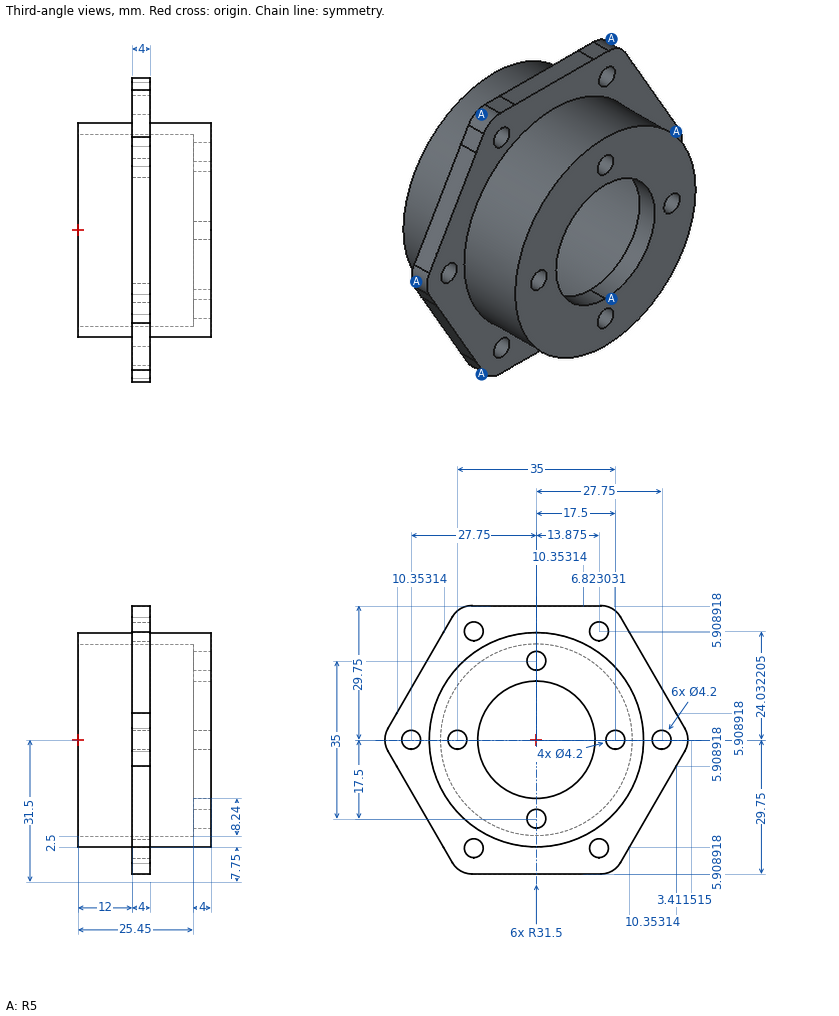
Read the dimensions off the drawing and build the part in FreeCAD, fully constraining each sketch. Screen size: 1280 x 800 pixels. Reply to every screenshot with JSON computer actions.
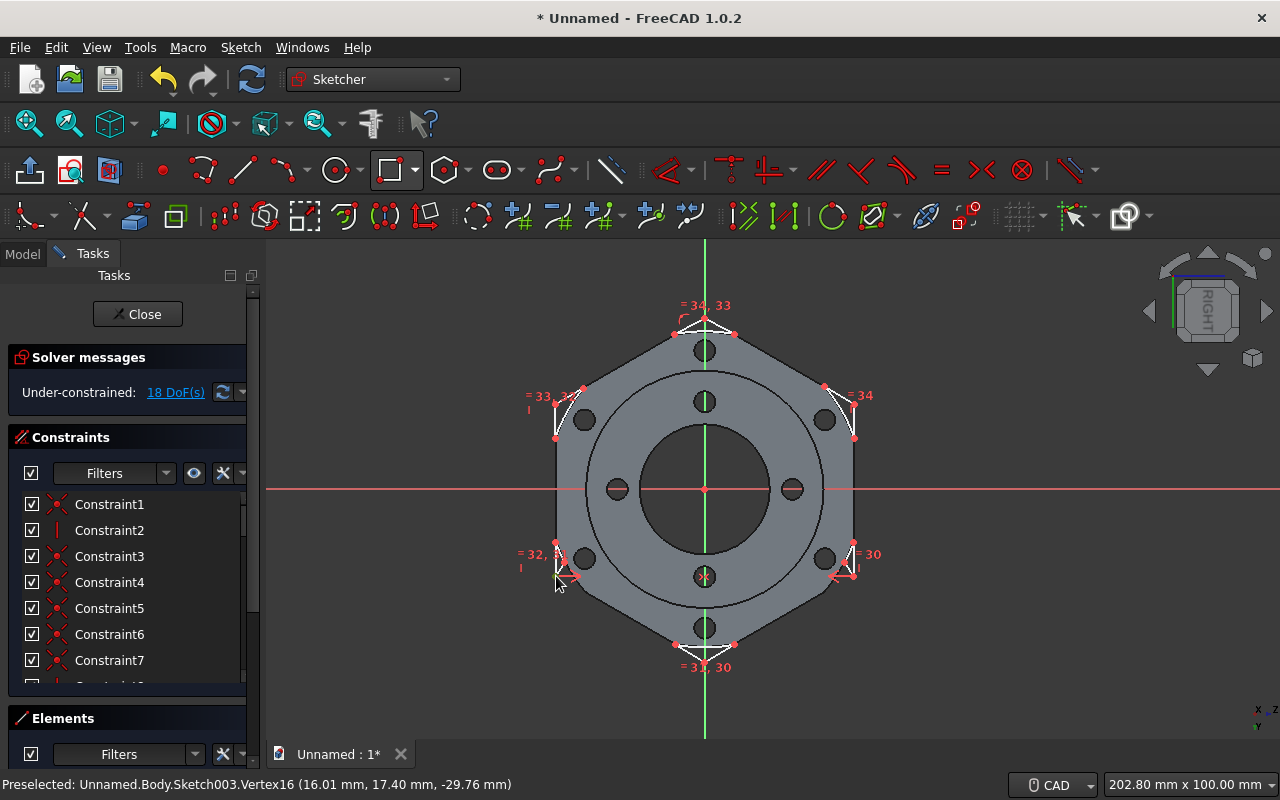
{"action": "left_click", "coordinate": [555, 405]}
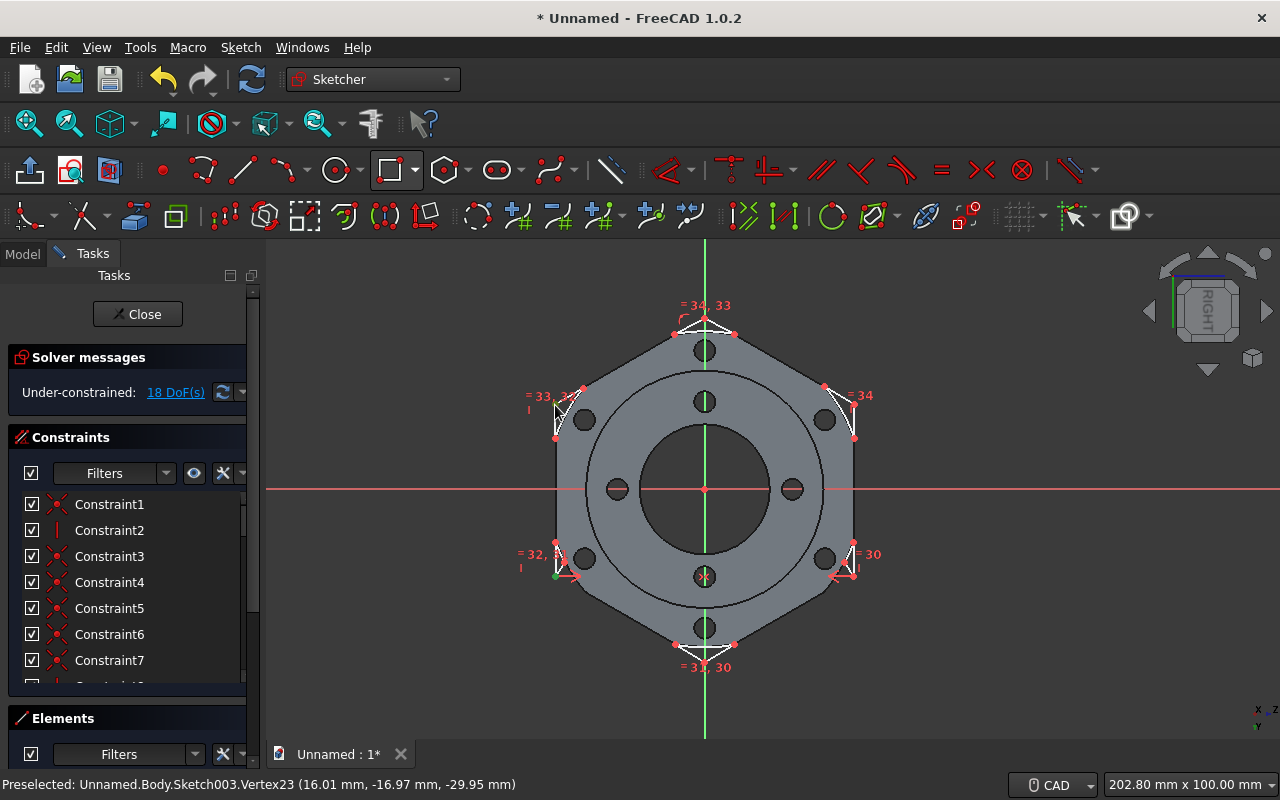
{"action": "left_click", "coordinate": [353, 489]}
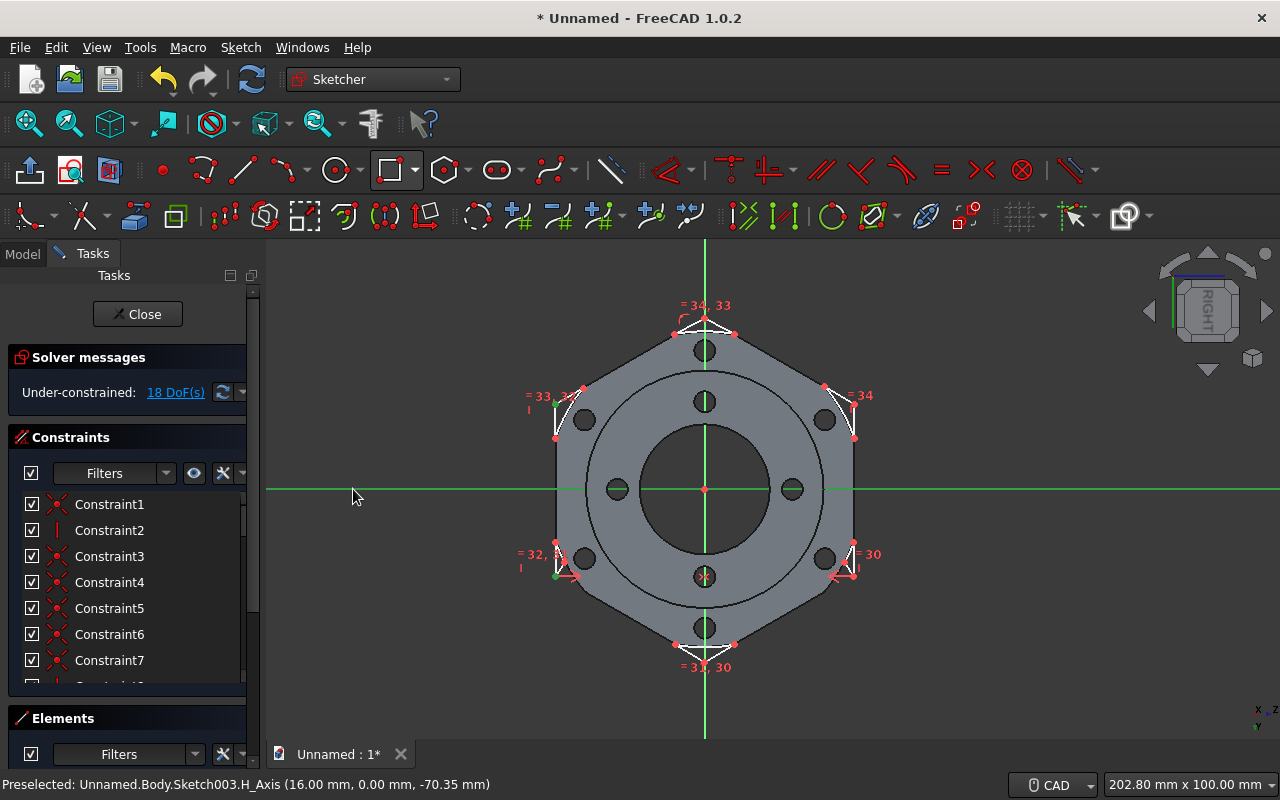
{"action": "left_click", "coordinate": [982, 170]}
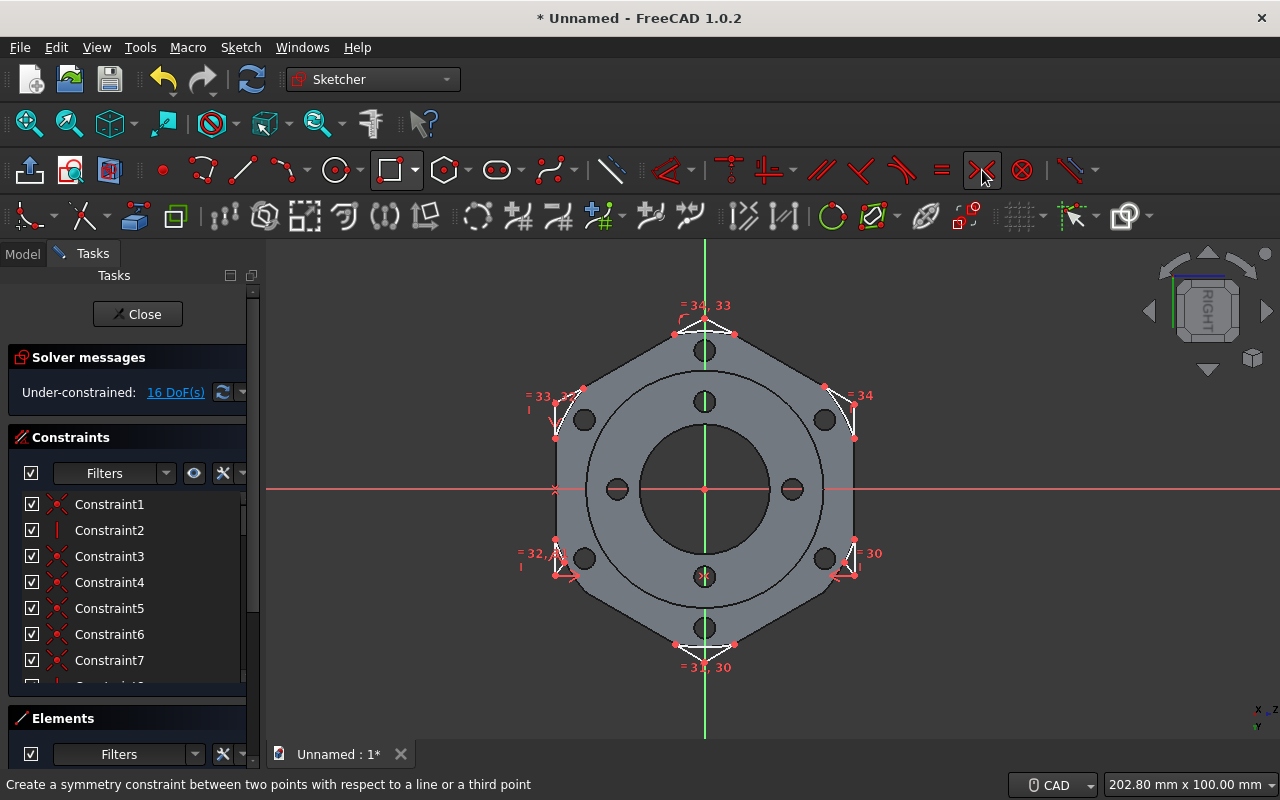
{"action": "left_click", "coordinate": [705, 663]}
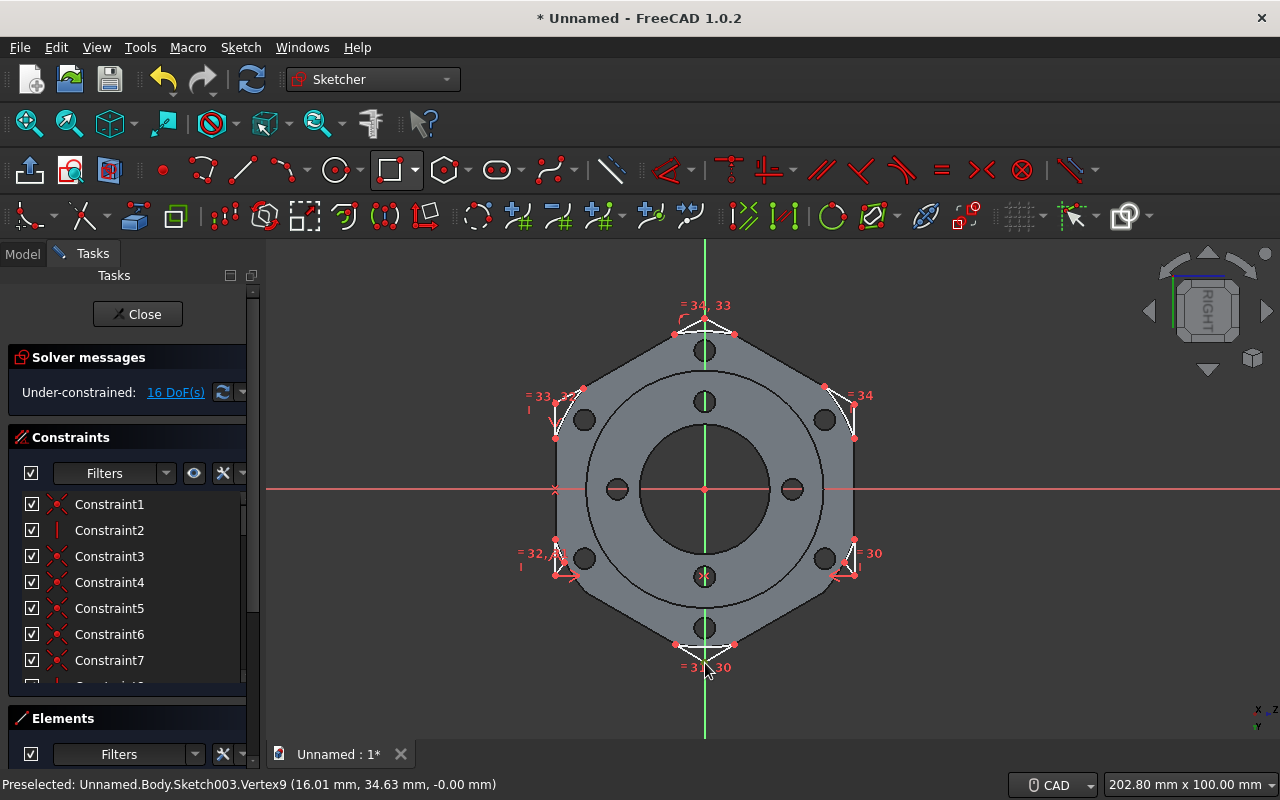
{"action": "left_click", "coordinate": [705, 318]}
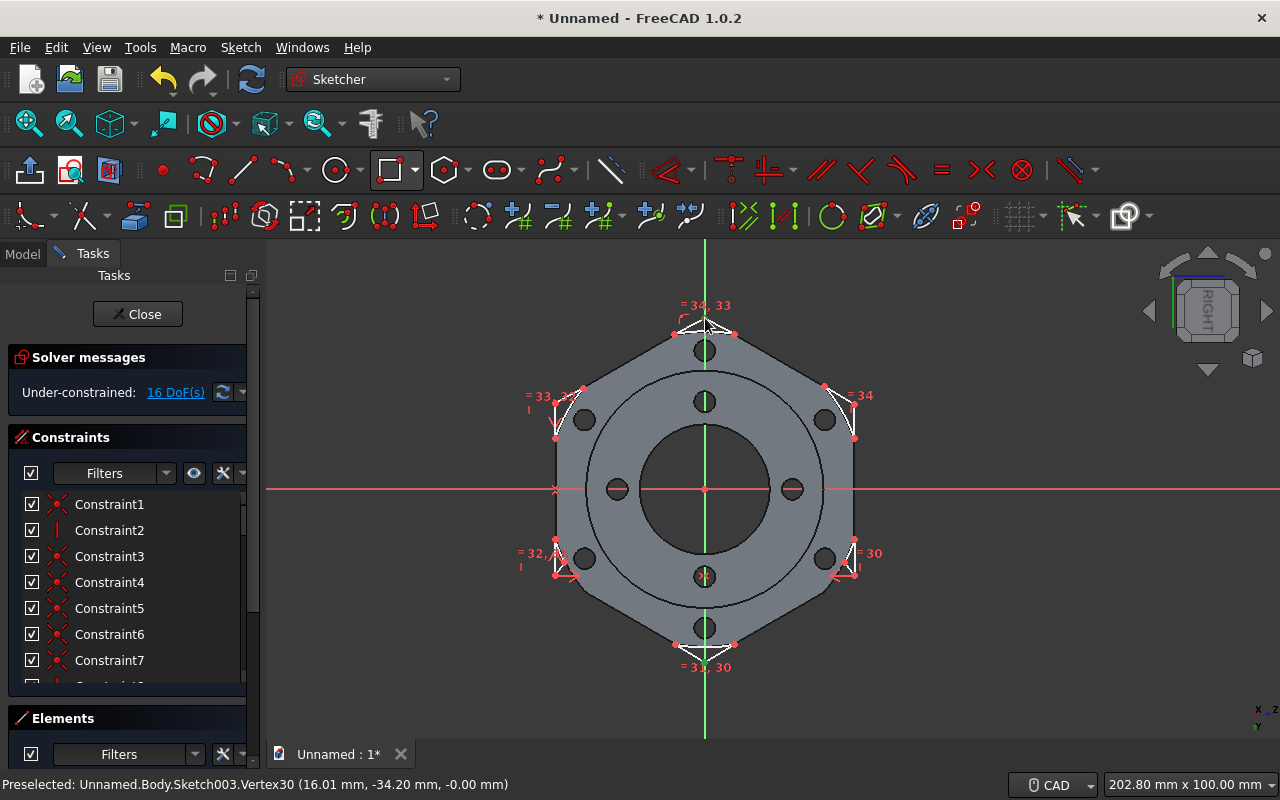
{"action": "left_click", "coordinate": [353, 489]}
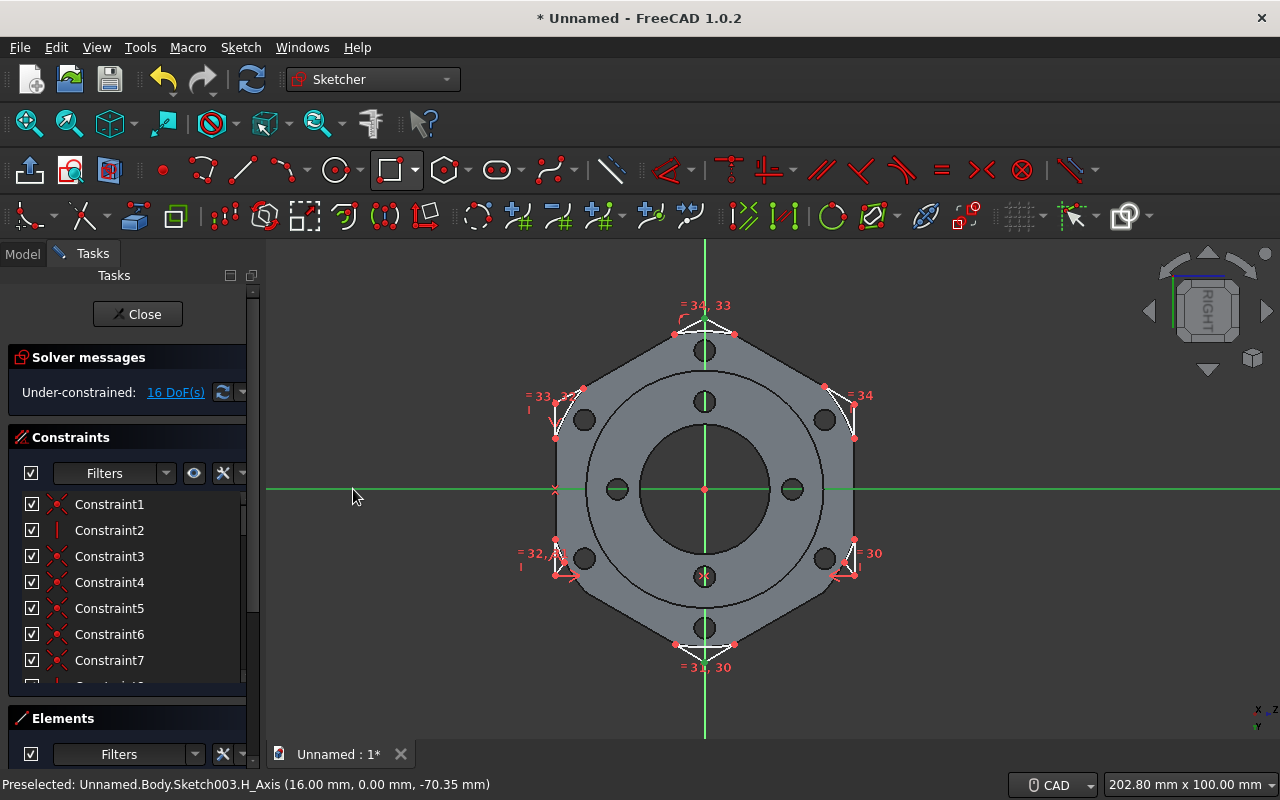
{"action": "key", "text": "s"}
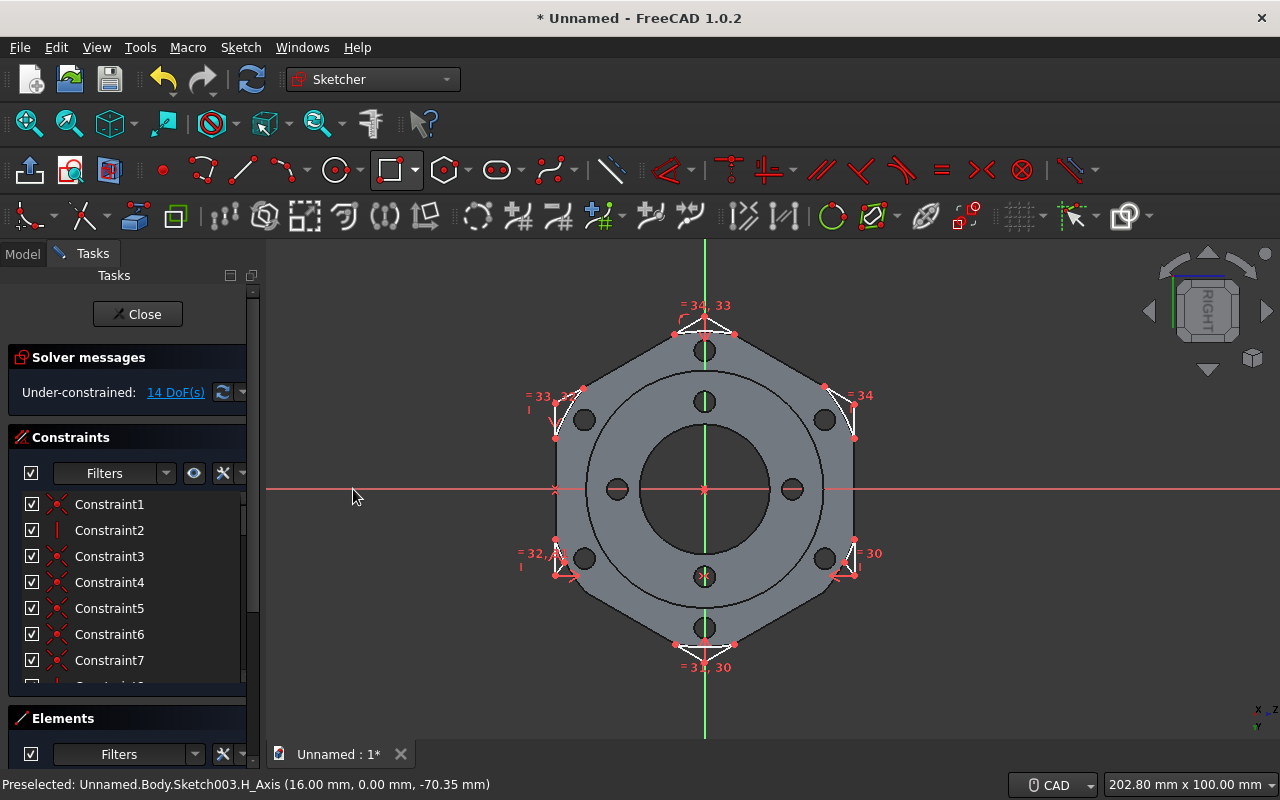
{"action": "left_click", "coordinate": [855, 576]}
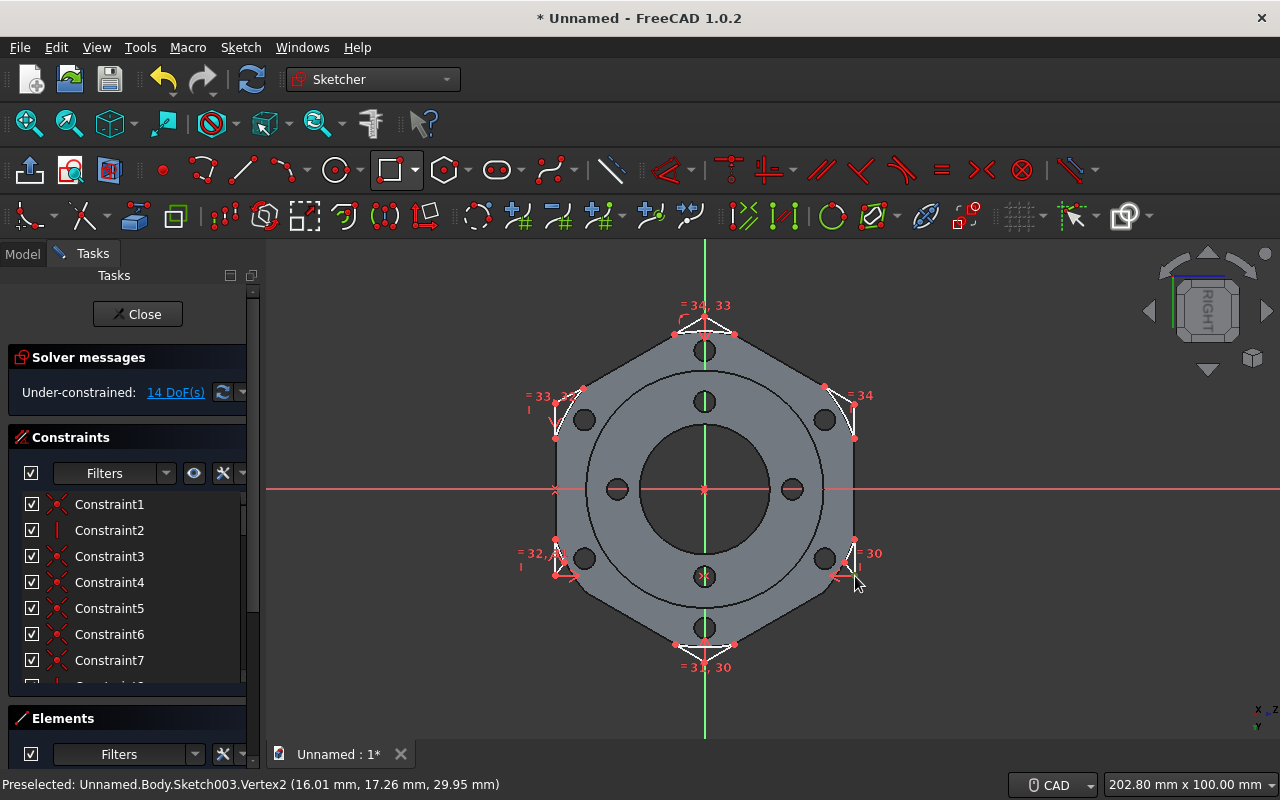
{"action": "scroll", "coordinate": [854, 404], "scroll_direction": "up", "scroll_amount": 4}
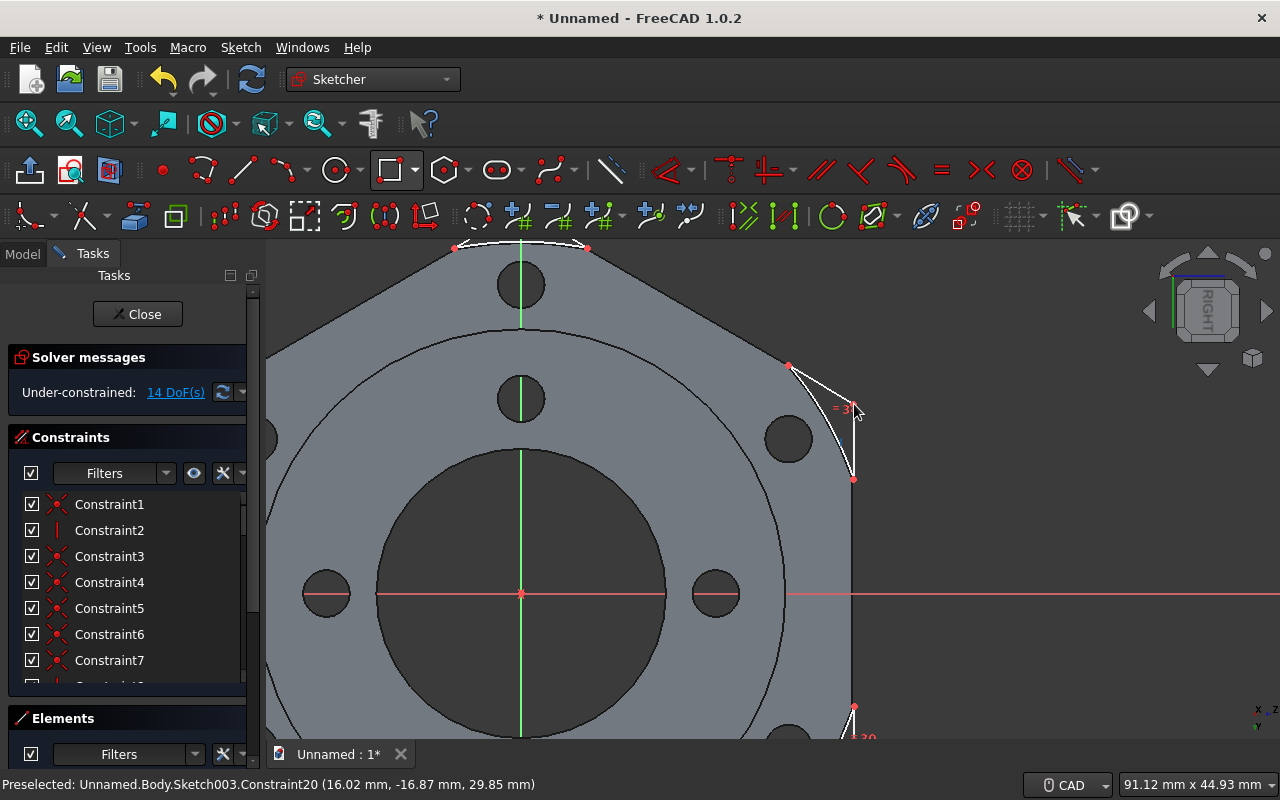
{"action": "scroll", "coordinate": [854, 404], "scroll_direction": "up", "scroll_amount": 4}